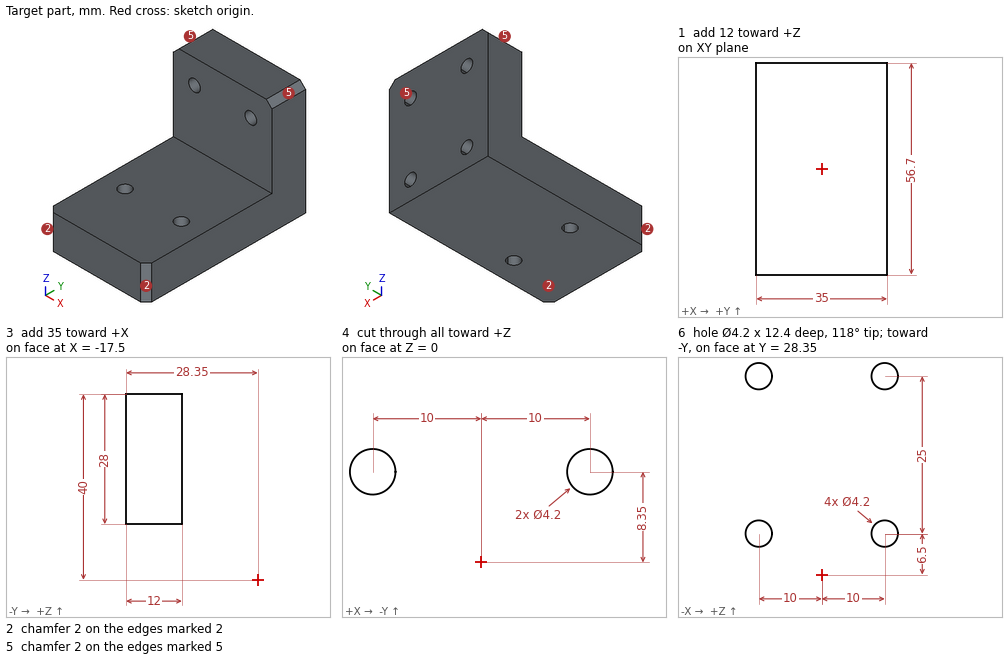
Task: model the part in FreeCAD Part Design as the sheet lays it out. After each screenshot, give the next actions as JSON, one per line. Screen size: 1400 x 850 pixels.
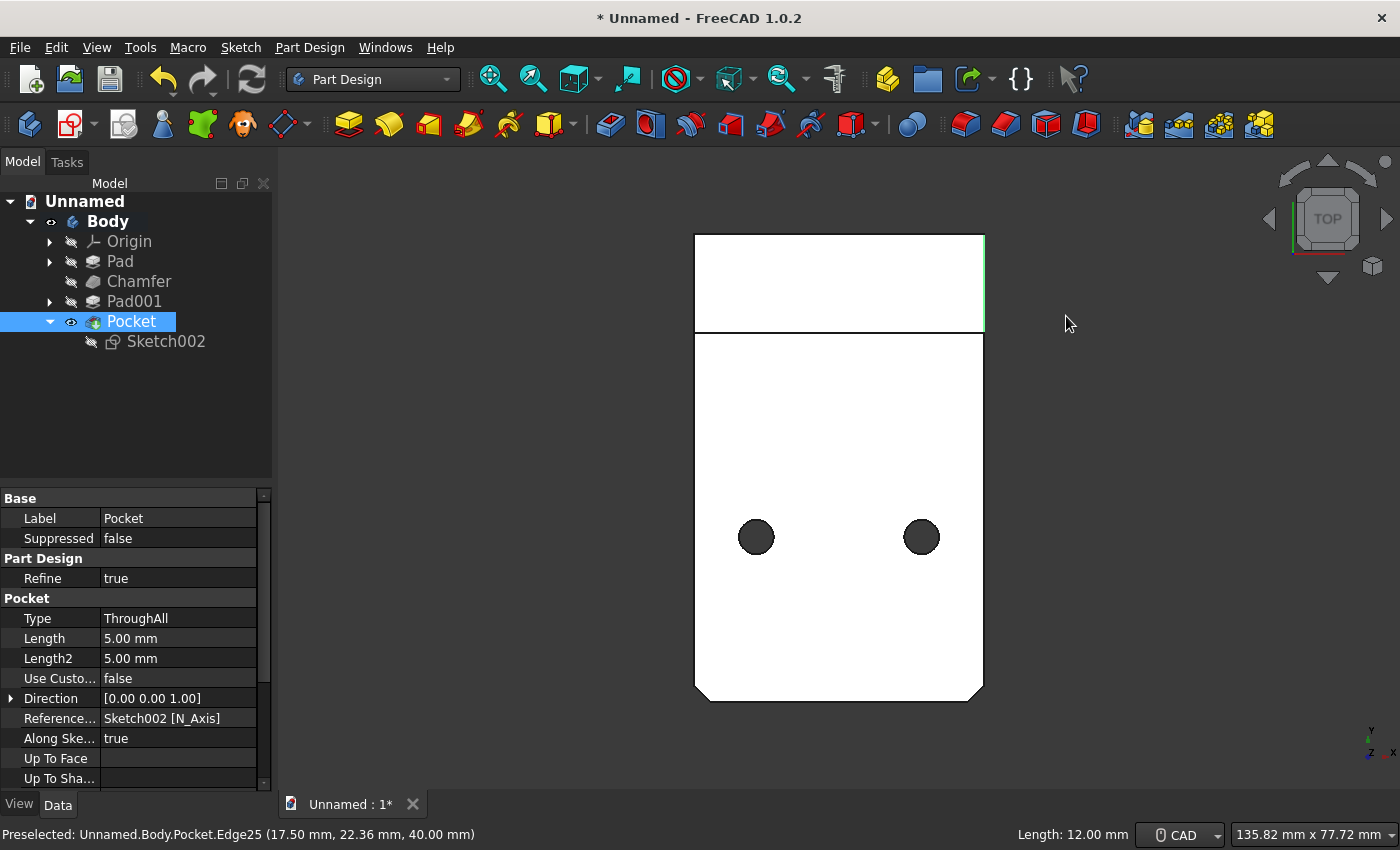
{"action": "left_click", "coordinate": [694, 282], "text": "ctrl"}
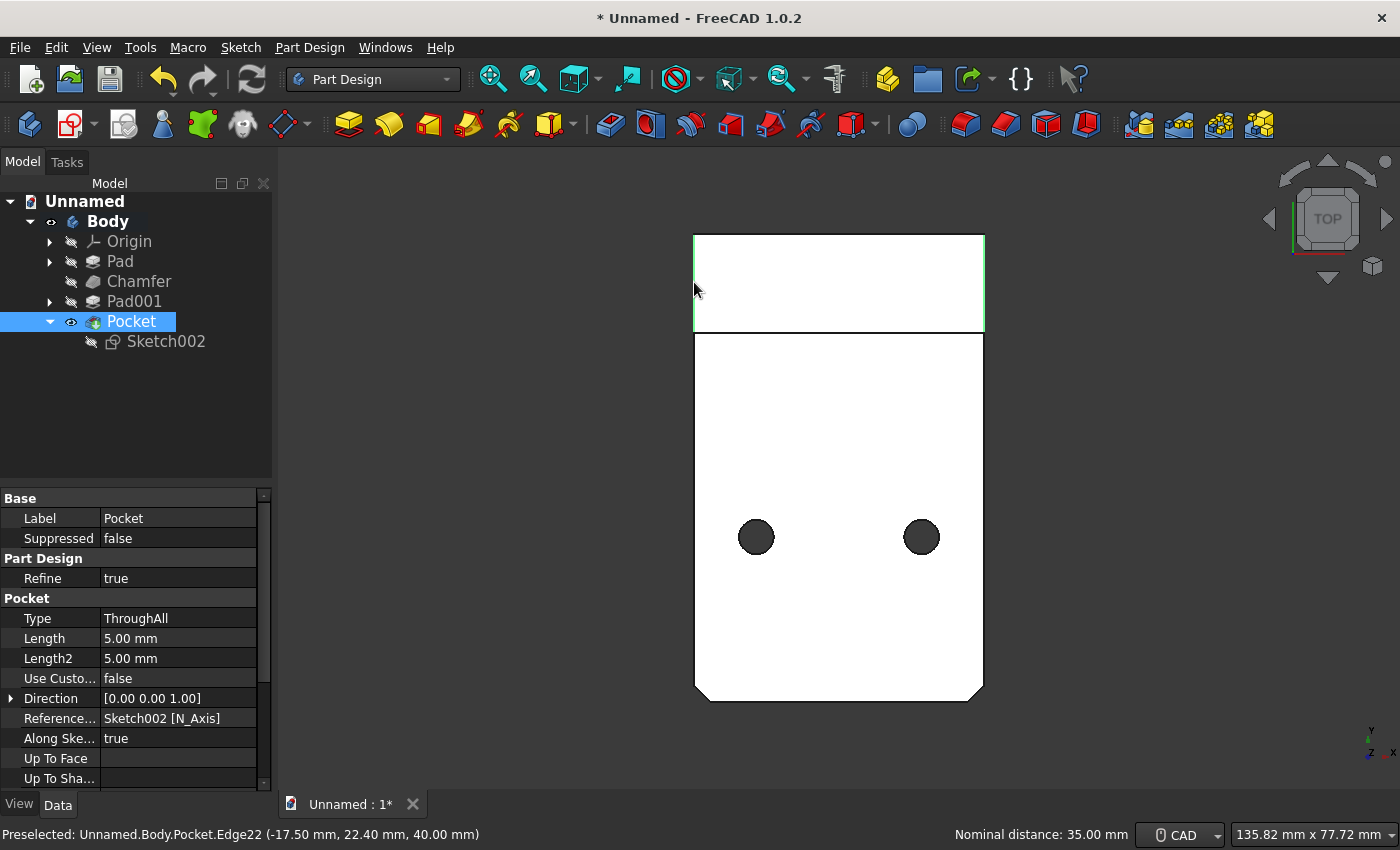
{"action": "left_click", "coordinate": [1006, 124]}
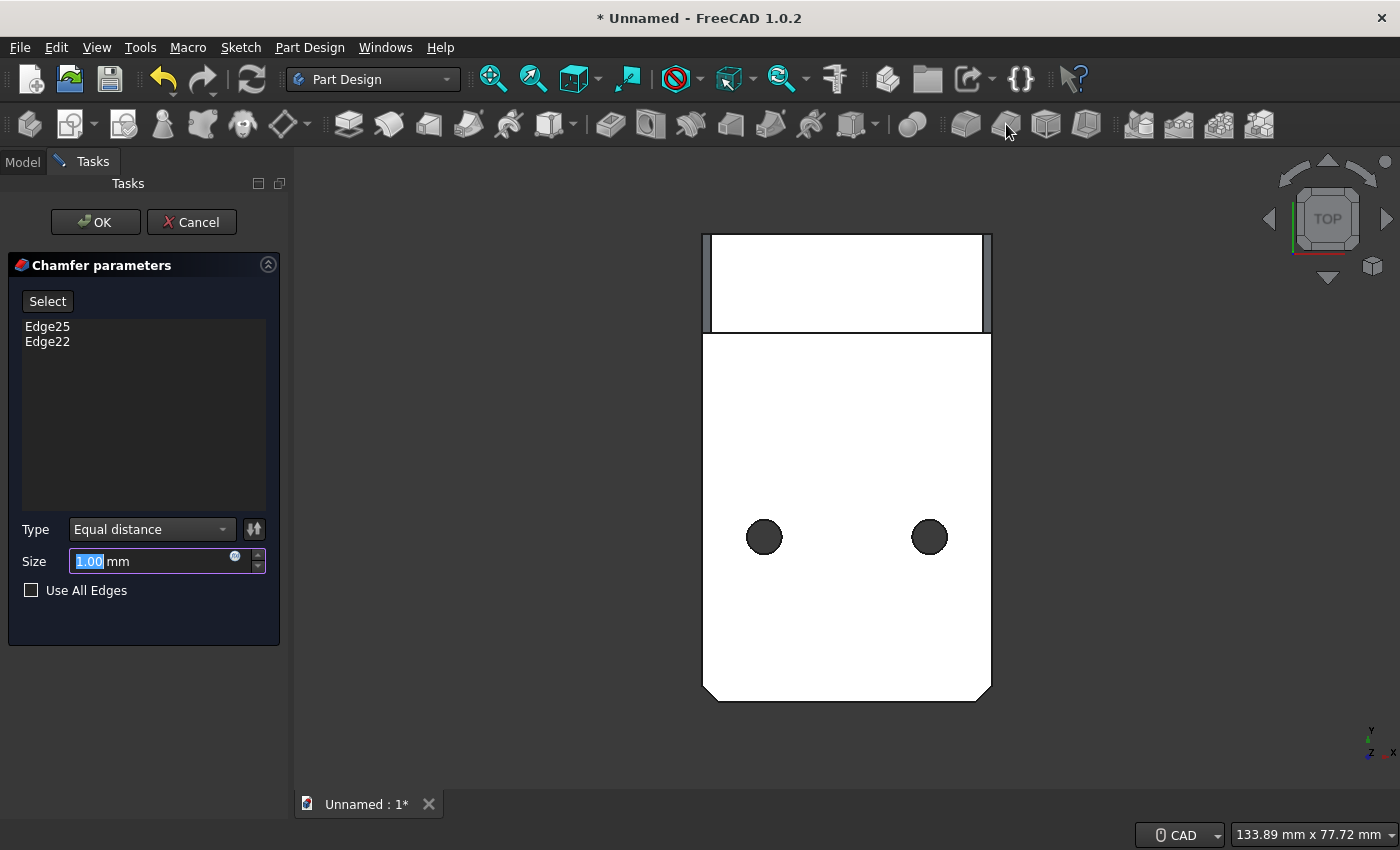
{"action": "type", "text": "2"}
{"action": "key", "text": "Tab"}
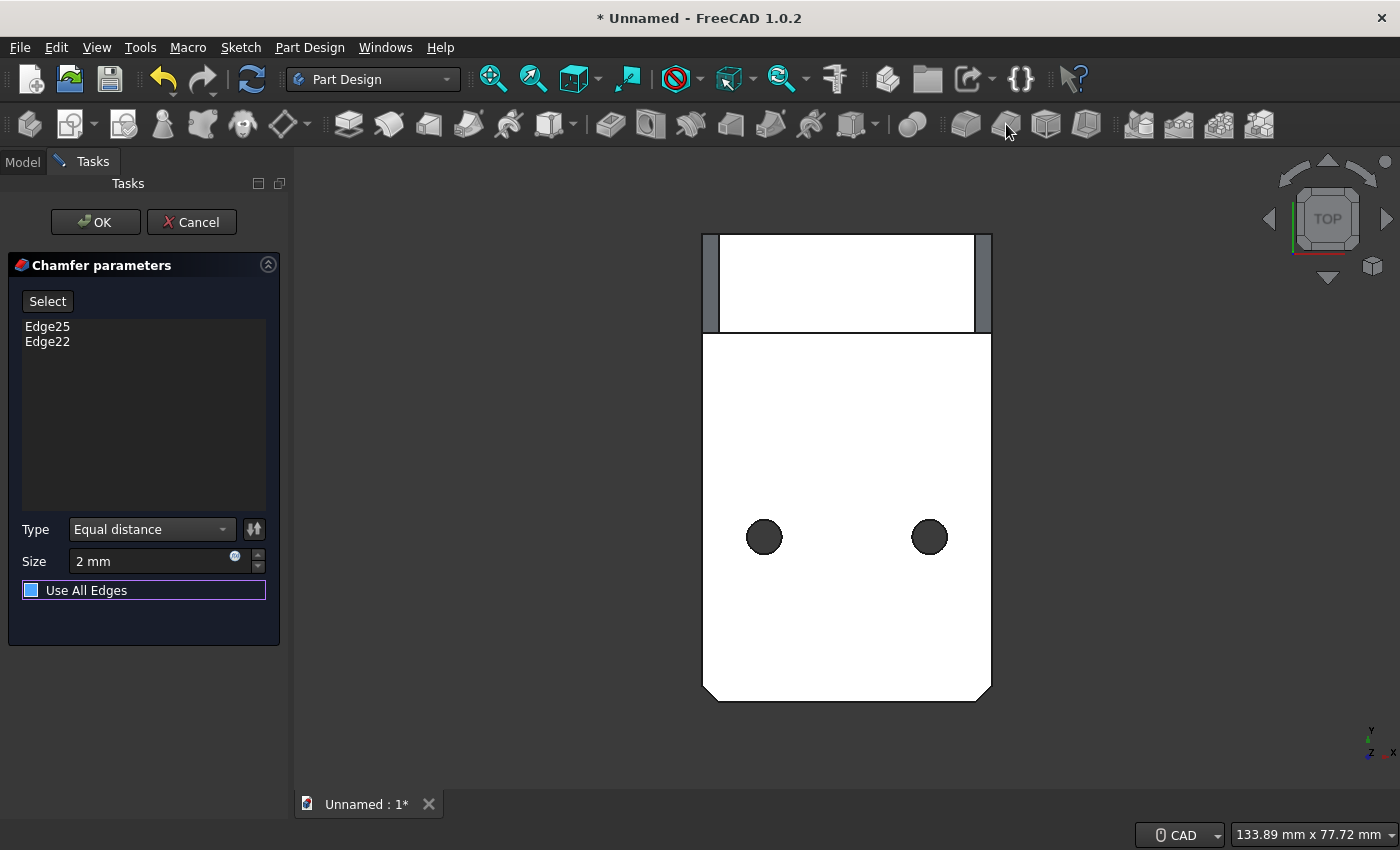
{"action": "left_click", "coordinate": [96, 222]}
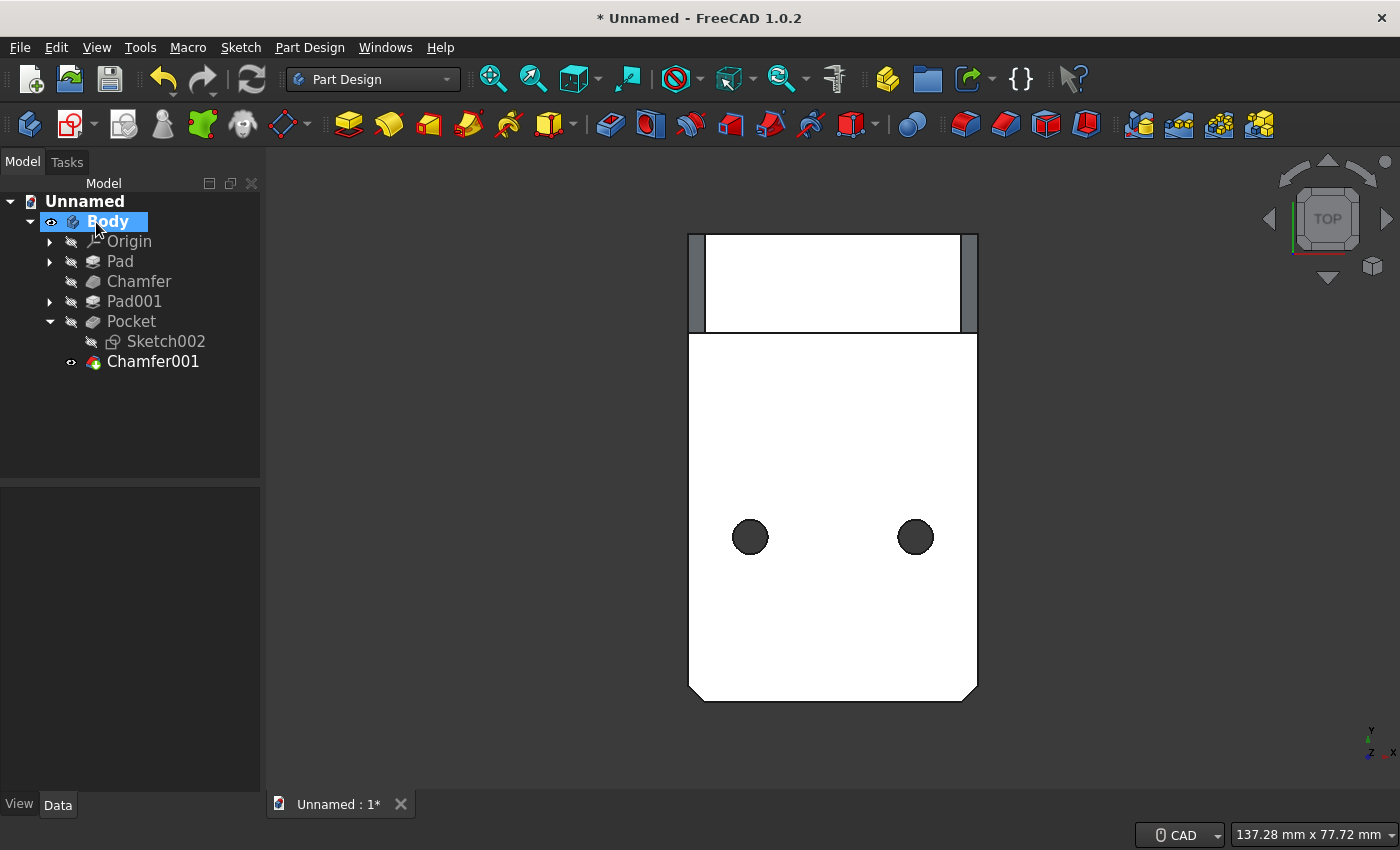
{"action": "key", "text": "4"}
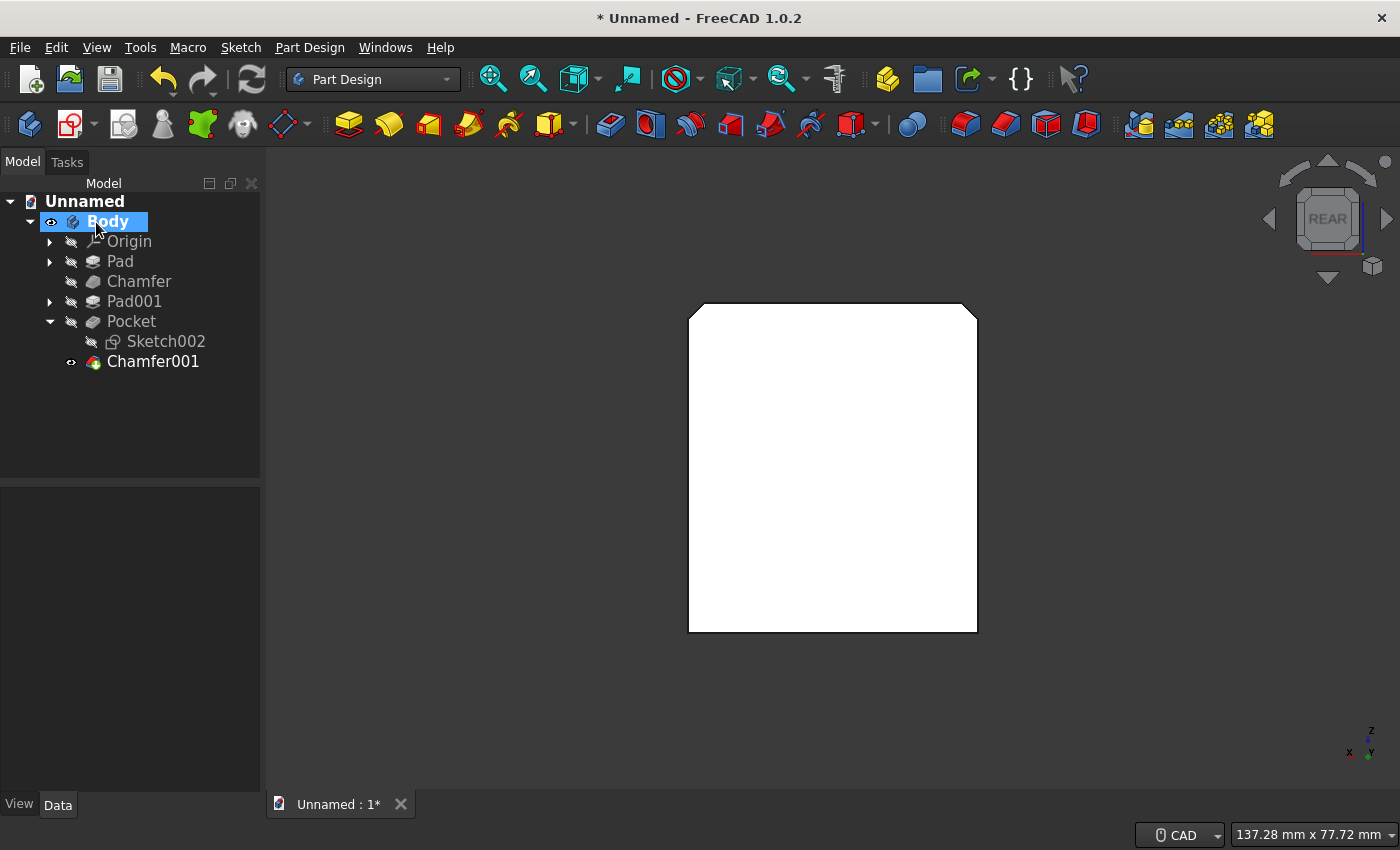
{"action": "left_click", "coordinate": [833, 467]}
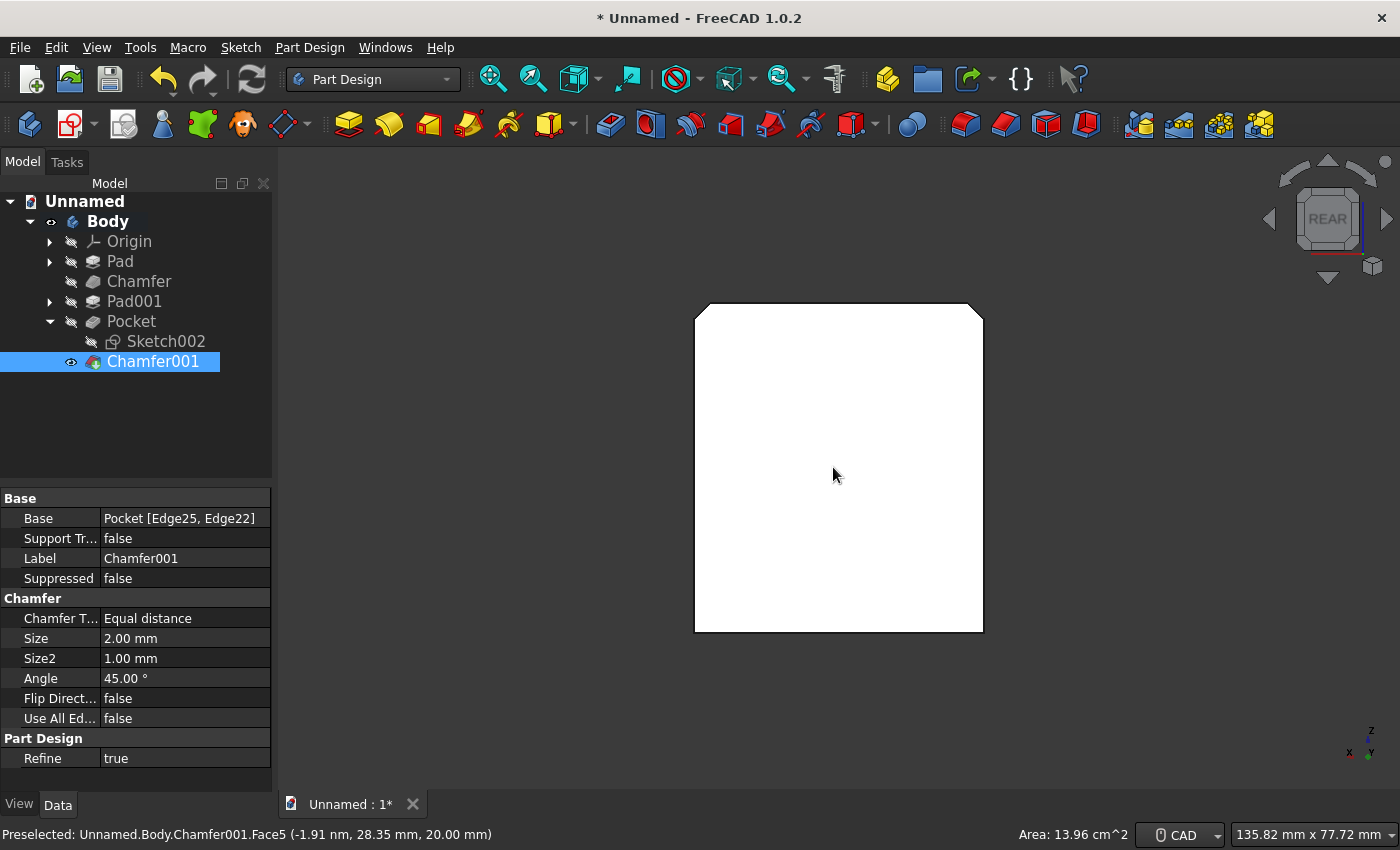
{"action": "left_click", "coordinate": [70, 124]}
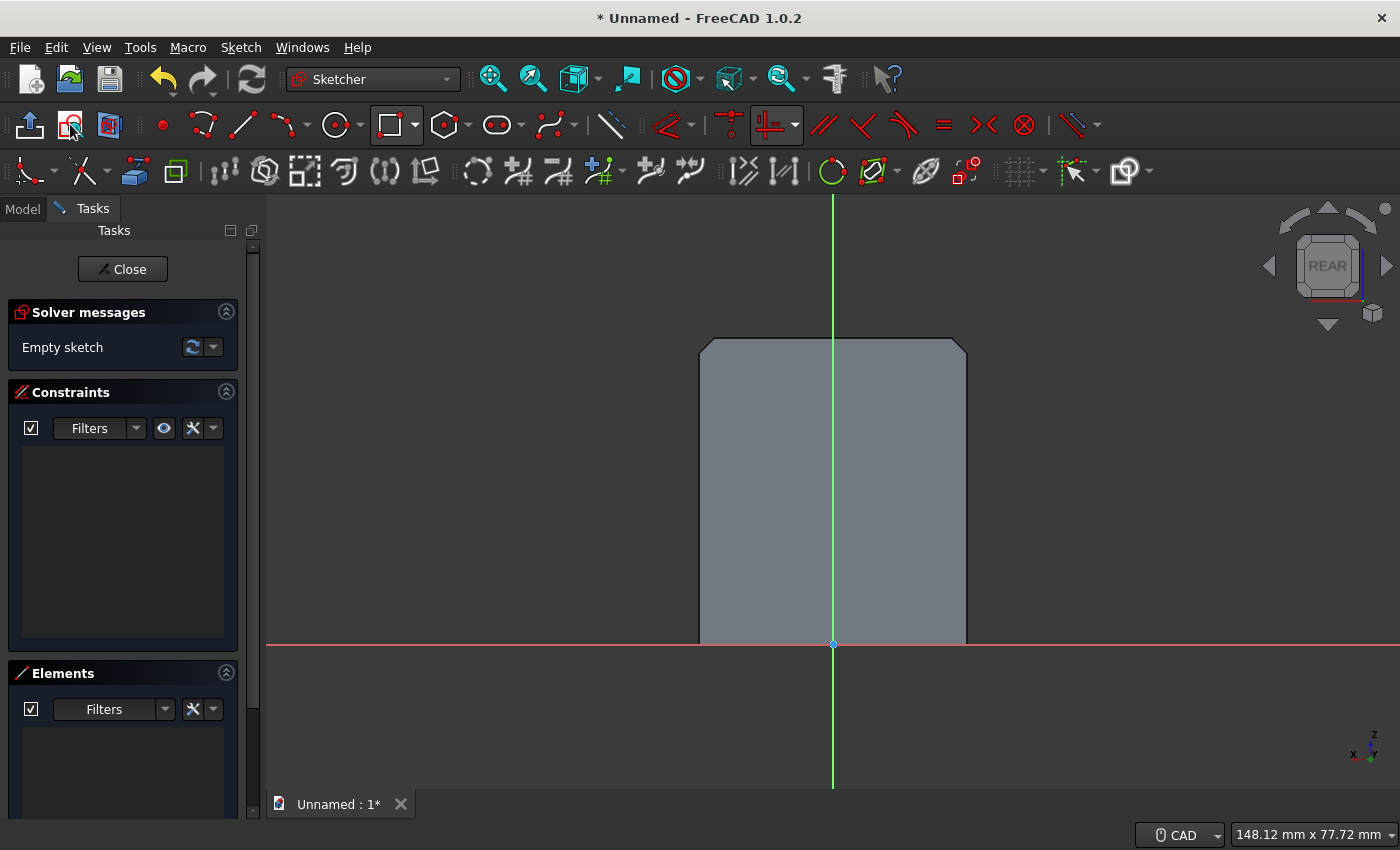
{"action": "scroll", "coordinate": [972, 566], "scroll_direction": "up", "scroll_amount": 2}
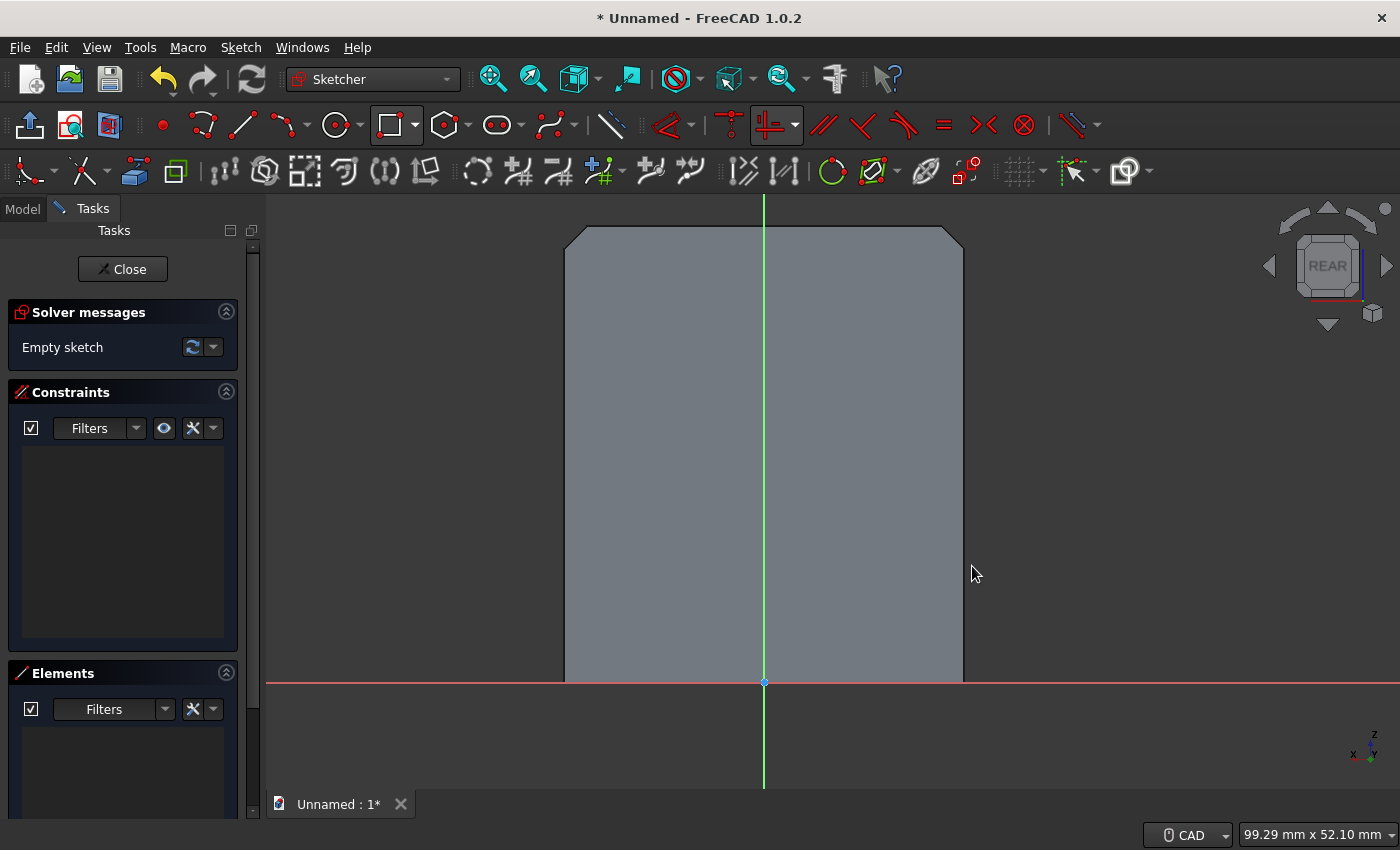
{"action": "left_click", "coordinate": [336, 126]}